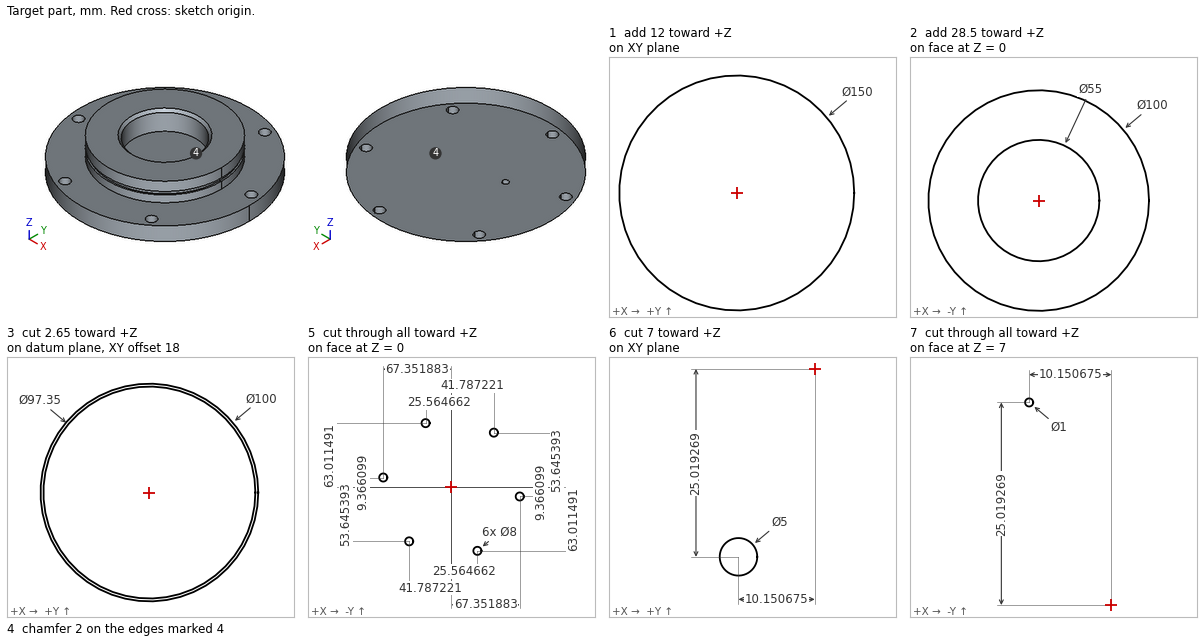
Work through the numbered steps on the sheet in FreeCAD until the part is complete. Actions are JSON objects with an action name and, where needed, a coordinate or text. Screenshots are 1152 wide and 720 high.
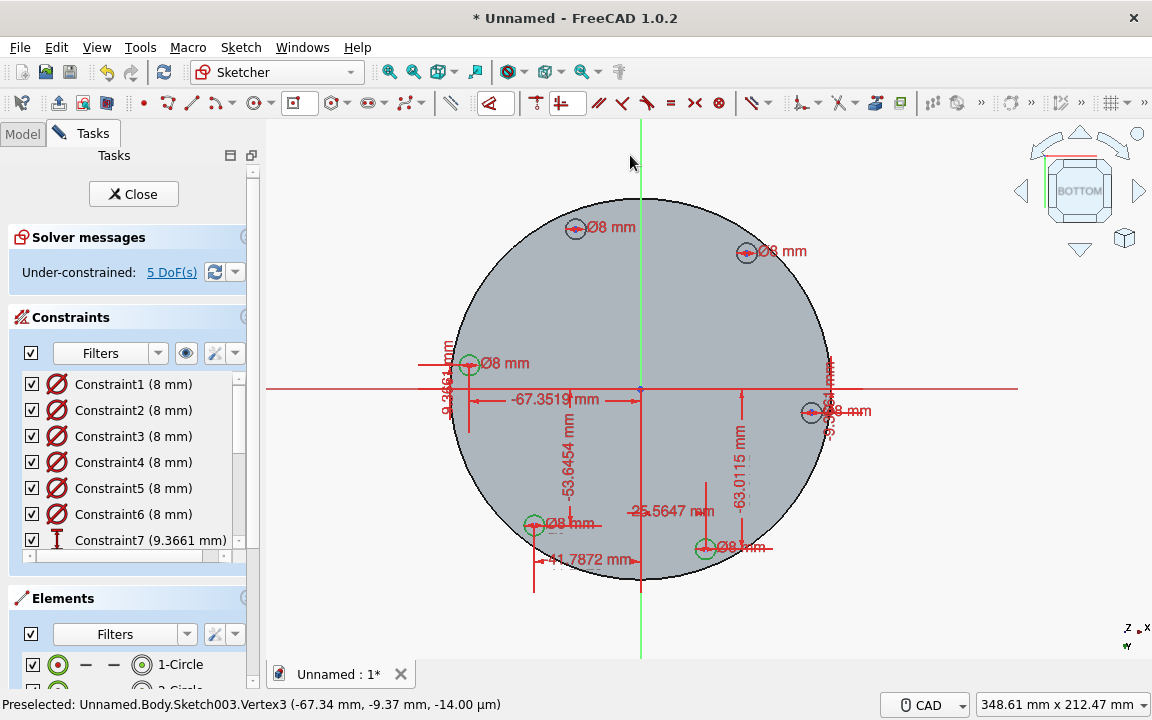
{"action": "left_click", "coordinate": [576, 229]}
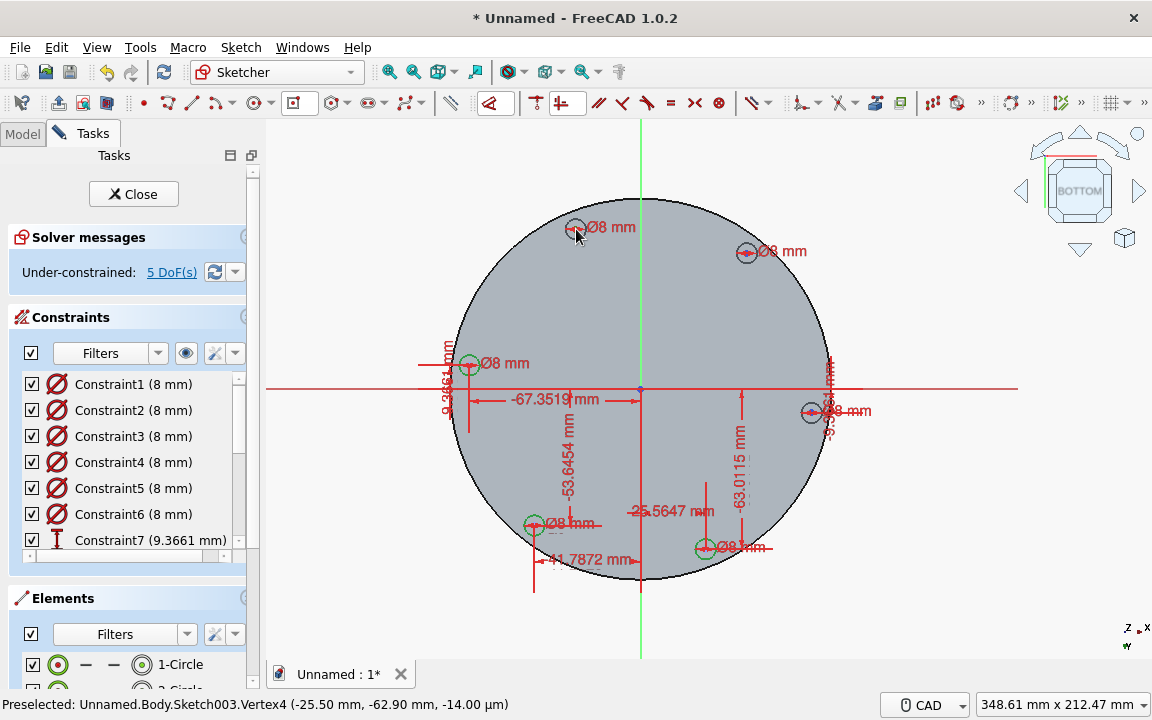
{"action": "key", "text": "l"}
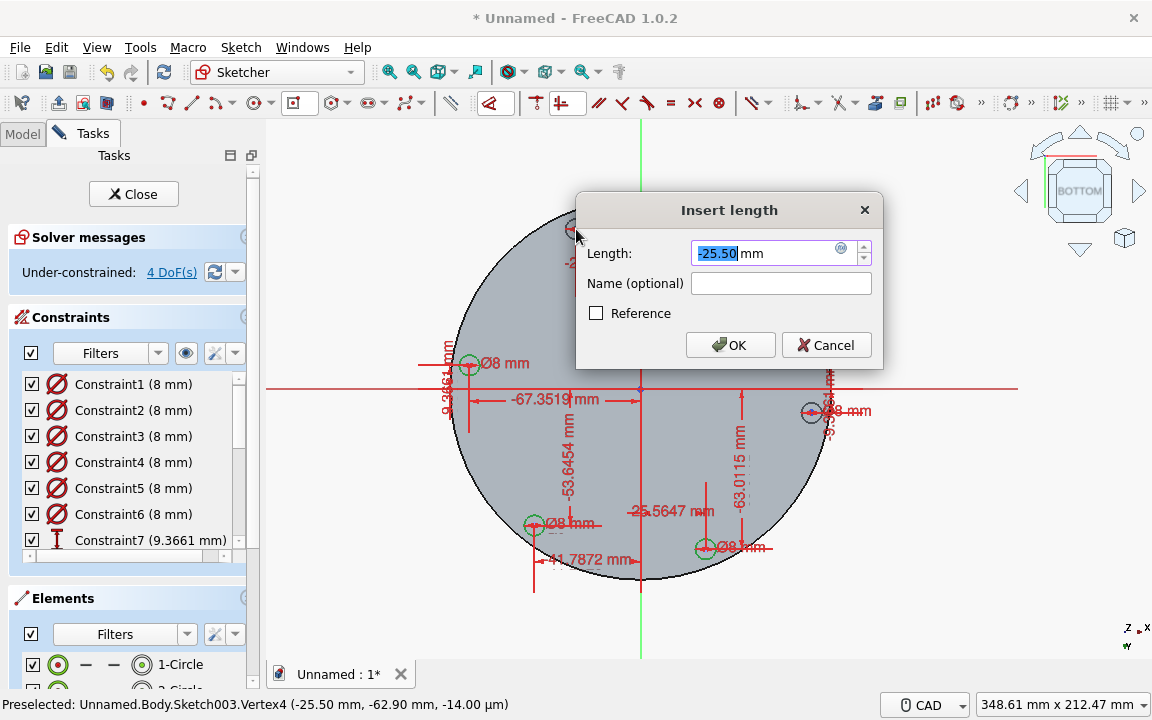
{"action": "type", "text": "-25.564662"}
{"action": "key", "text": "Return"}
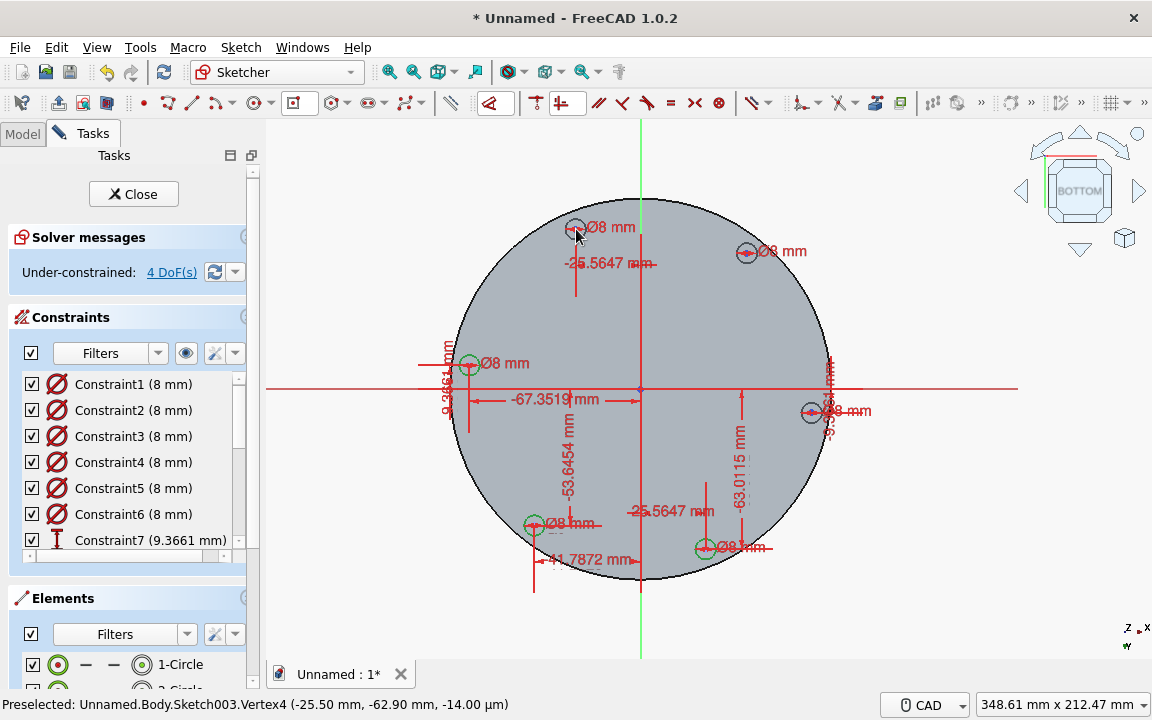
{"action": "left_click", "coordinate": [576, 229]}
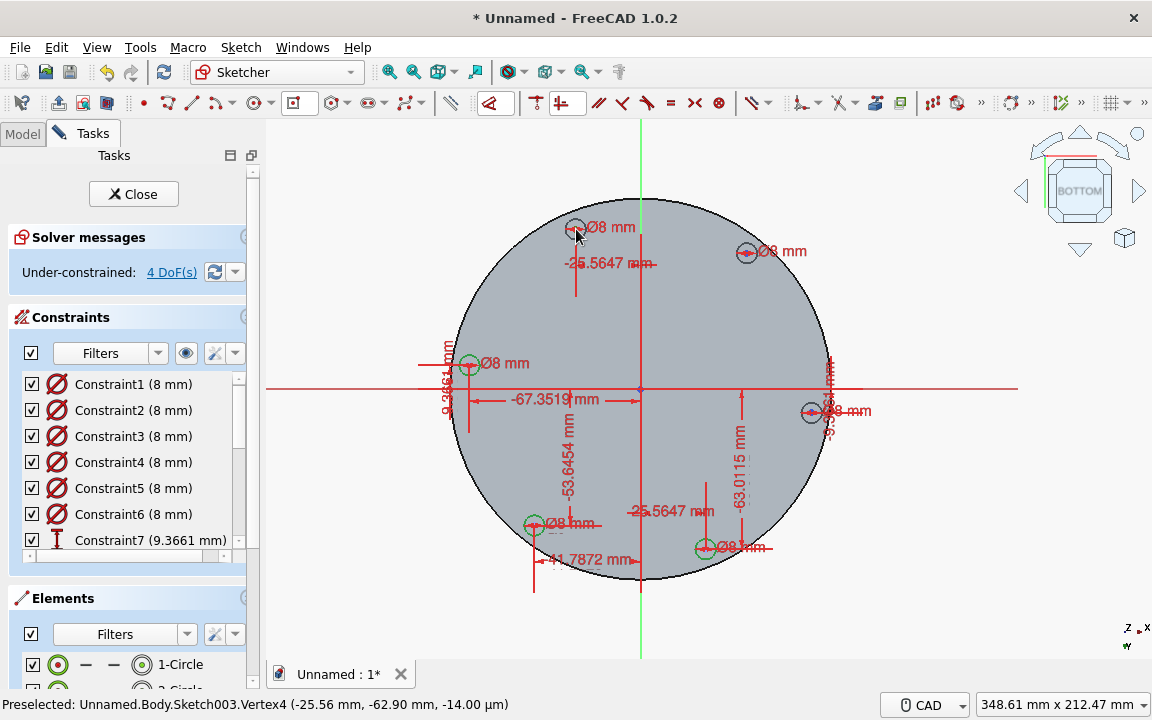
{"action": "key", "text": "i"}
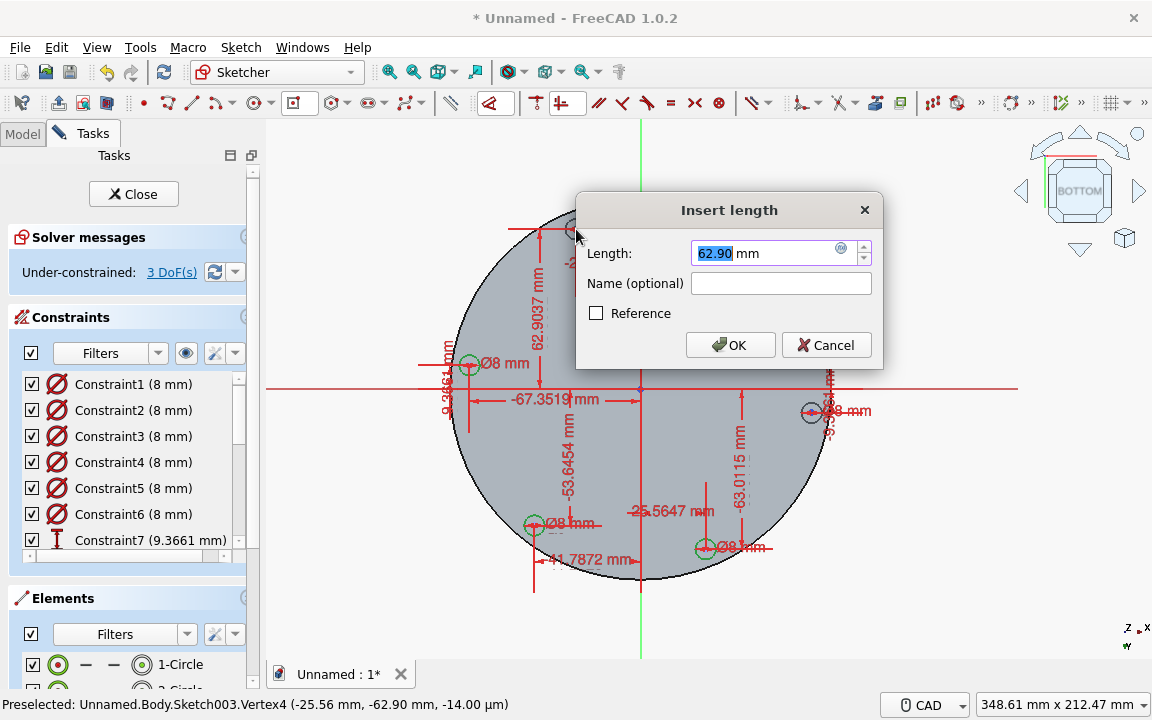
{"action": "type", "text": "63.011491"}
{"action": "key", "text": "Return"}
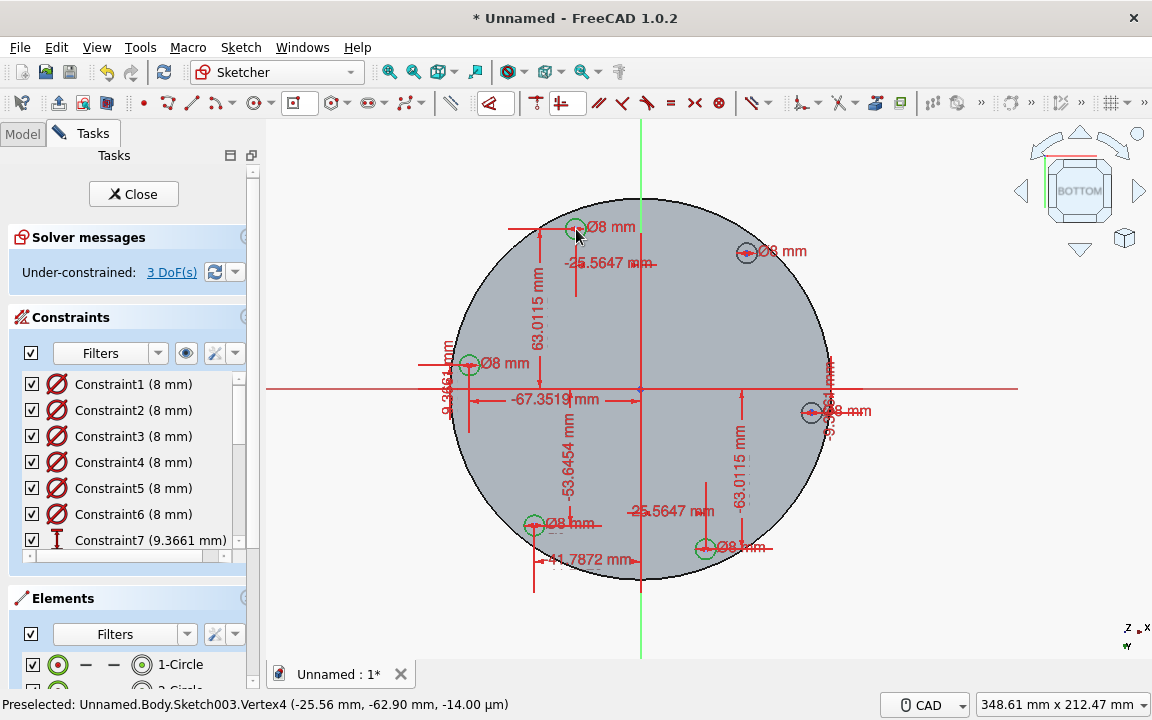
{"action": "left_click", "coordinate": [747, 253]}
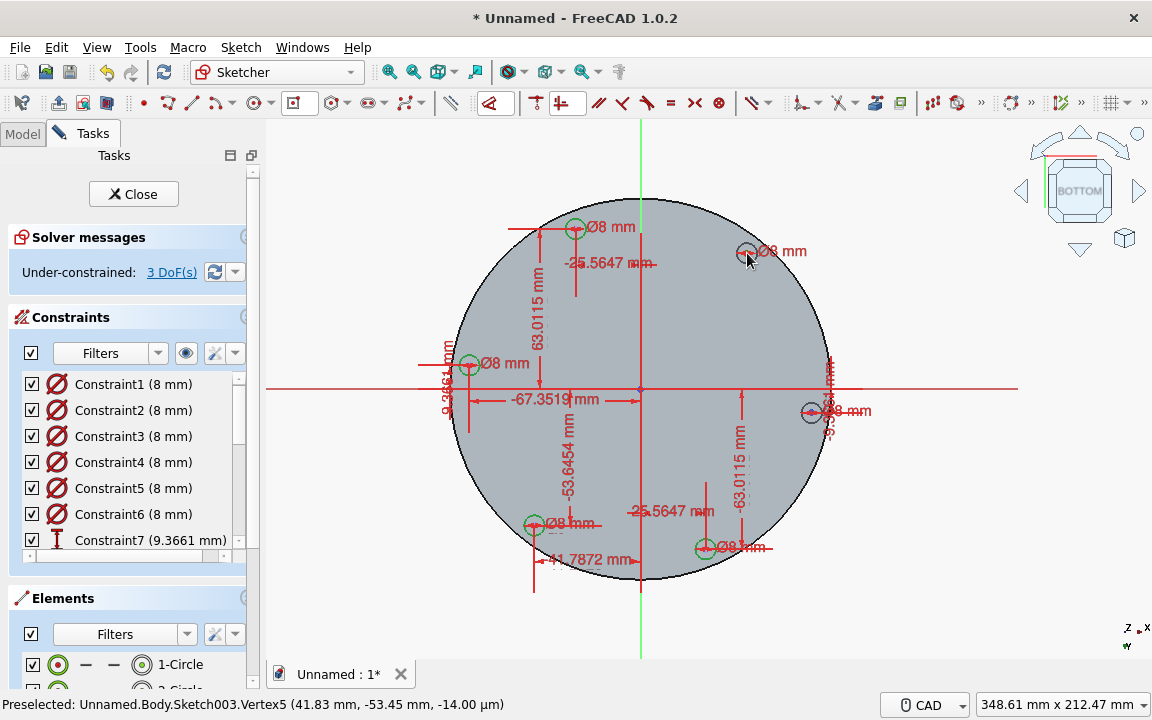
{"action": "key", "text": "l"}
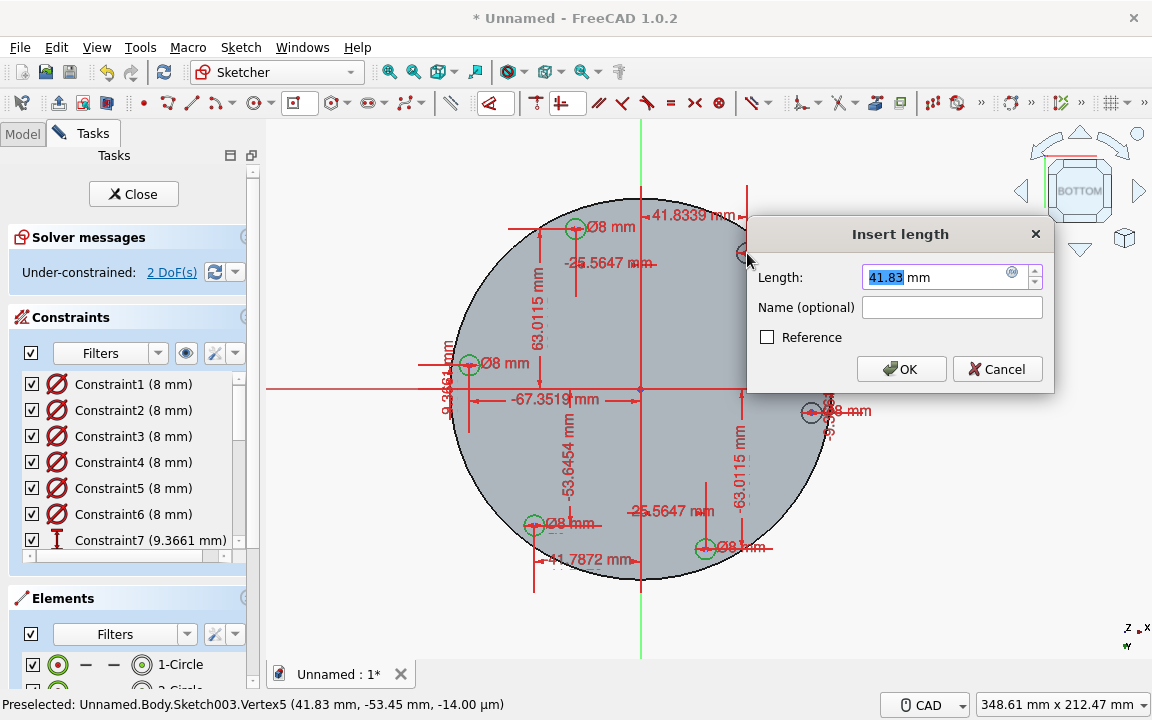
{"action": "type", "text": "41.787221"}
{"action": "key", "text": "Return"}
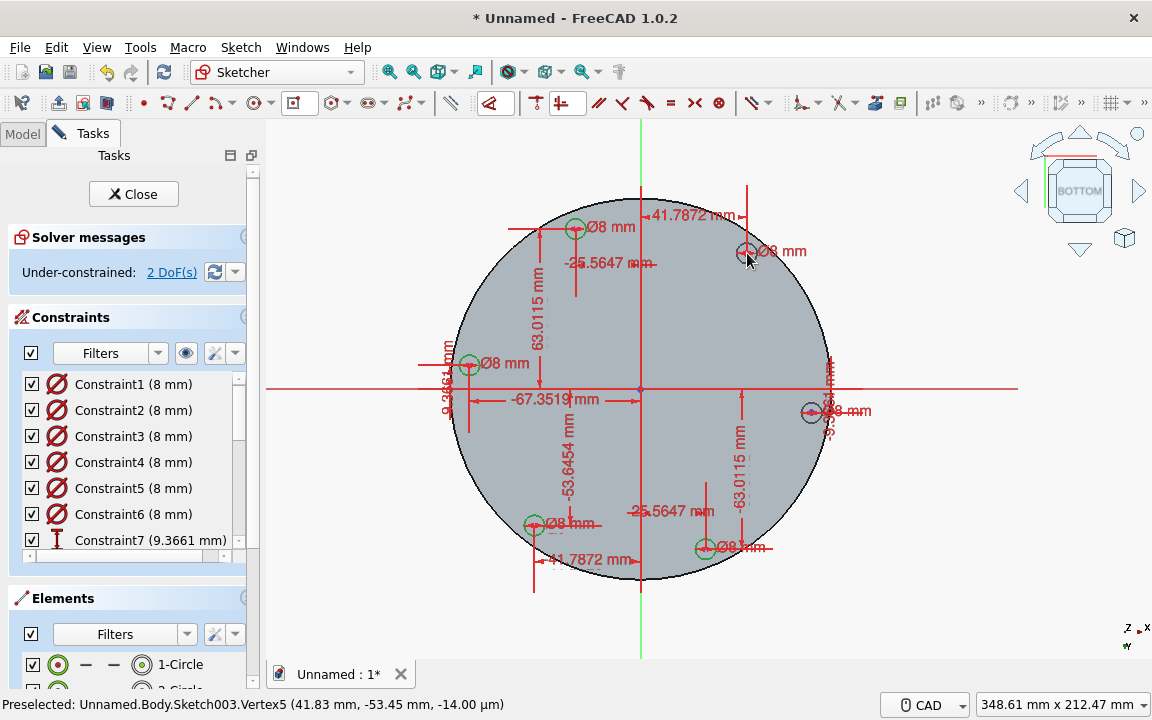
{"action": "left_click", "coordinate": [747, 253]}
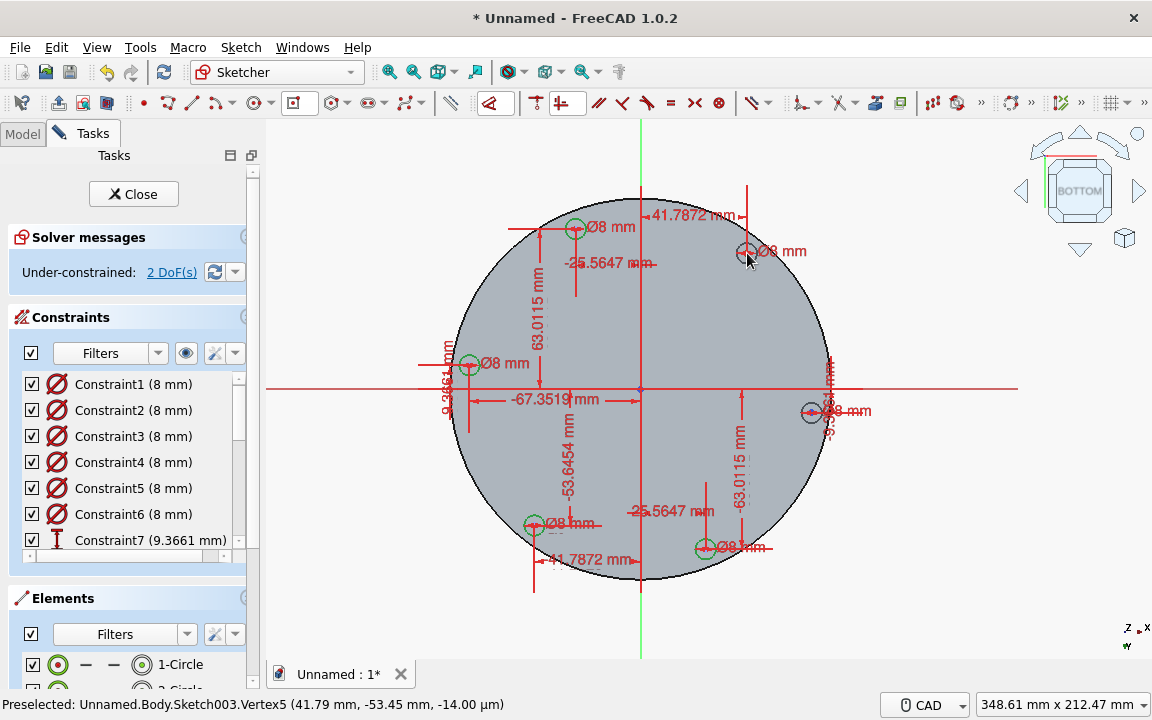
{"action": "left_click", "coordinate": [508, 104]}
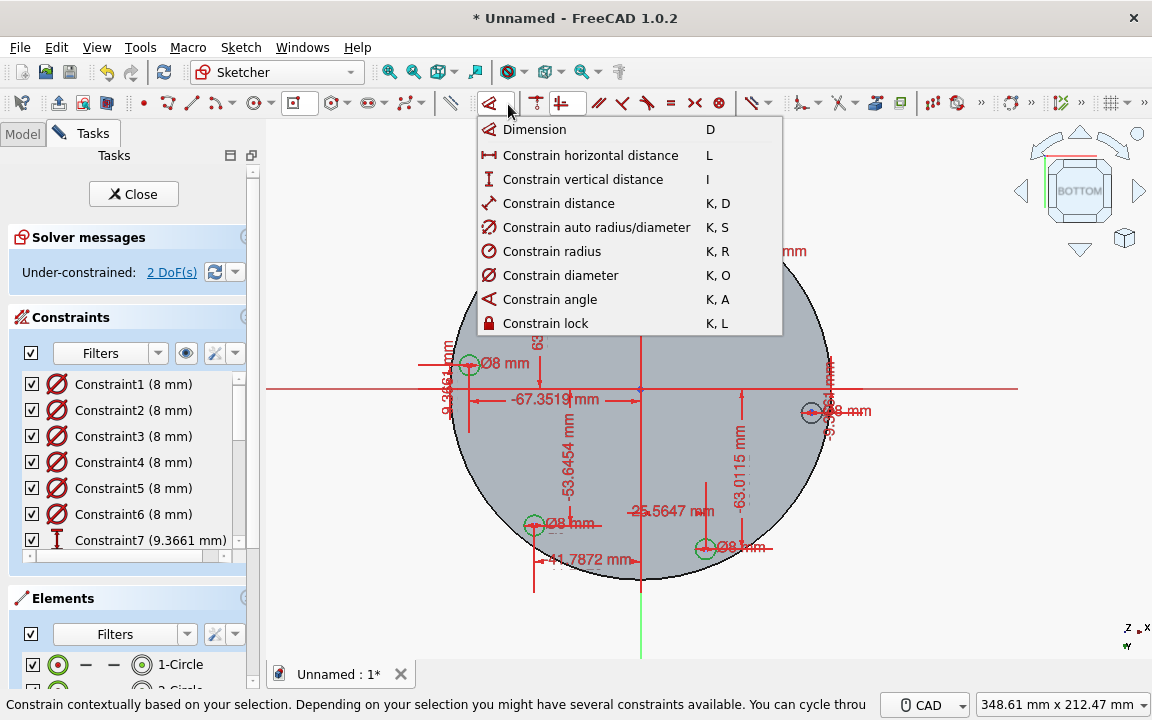
{"action": "left_click", "coordinate": [630, 179]}